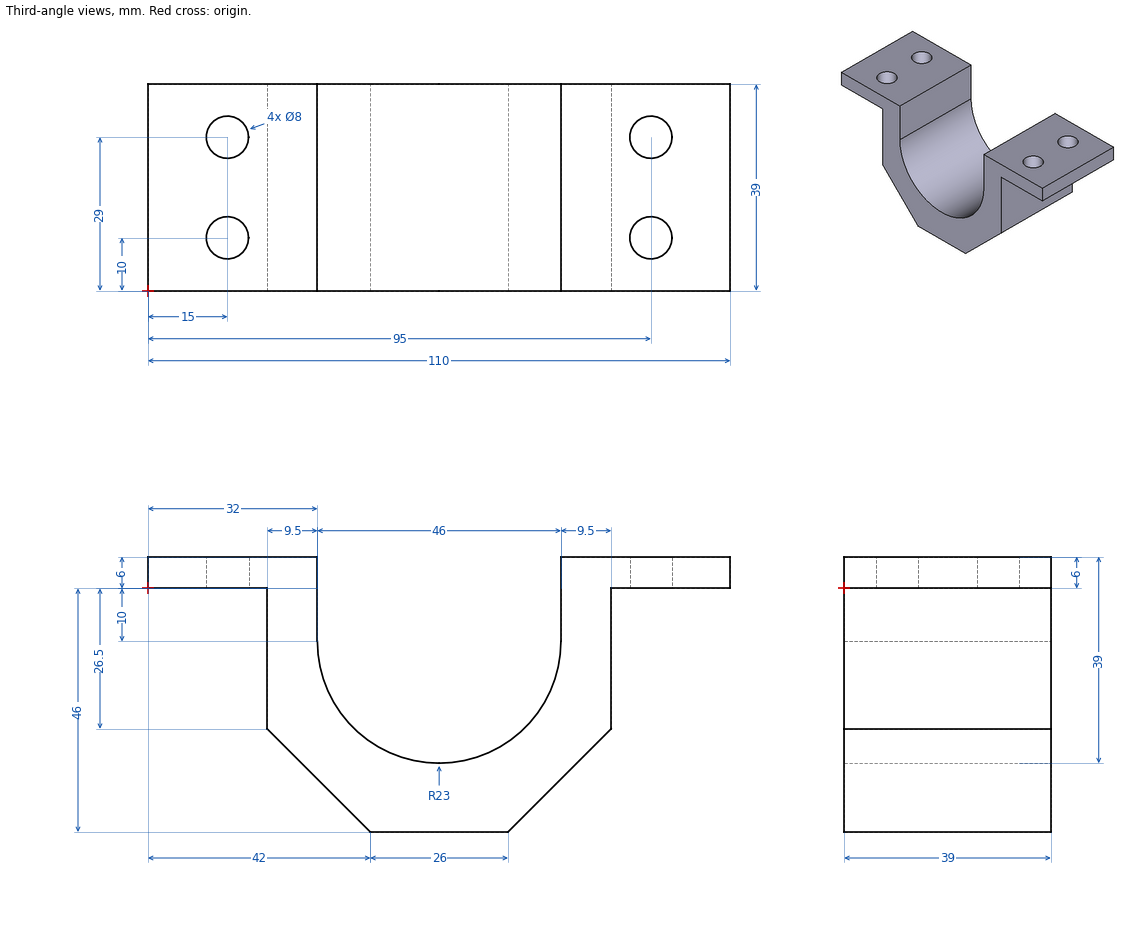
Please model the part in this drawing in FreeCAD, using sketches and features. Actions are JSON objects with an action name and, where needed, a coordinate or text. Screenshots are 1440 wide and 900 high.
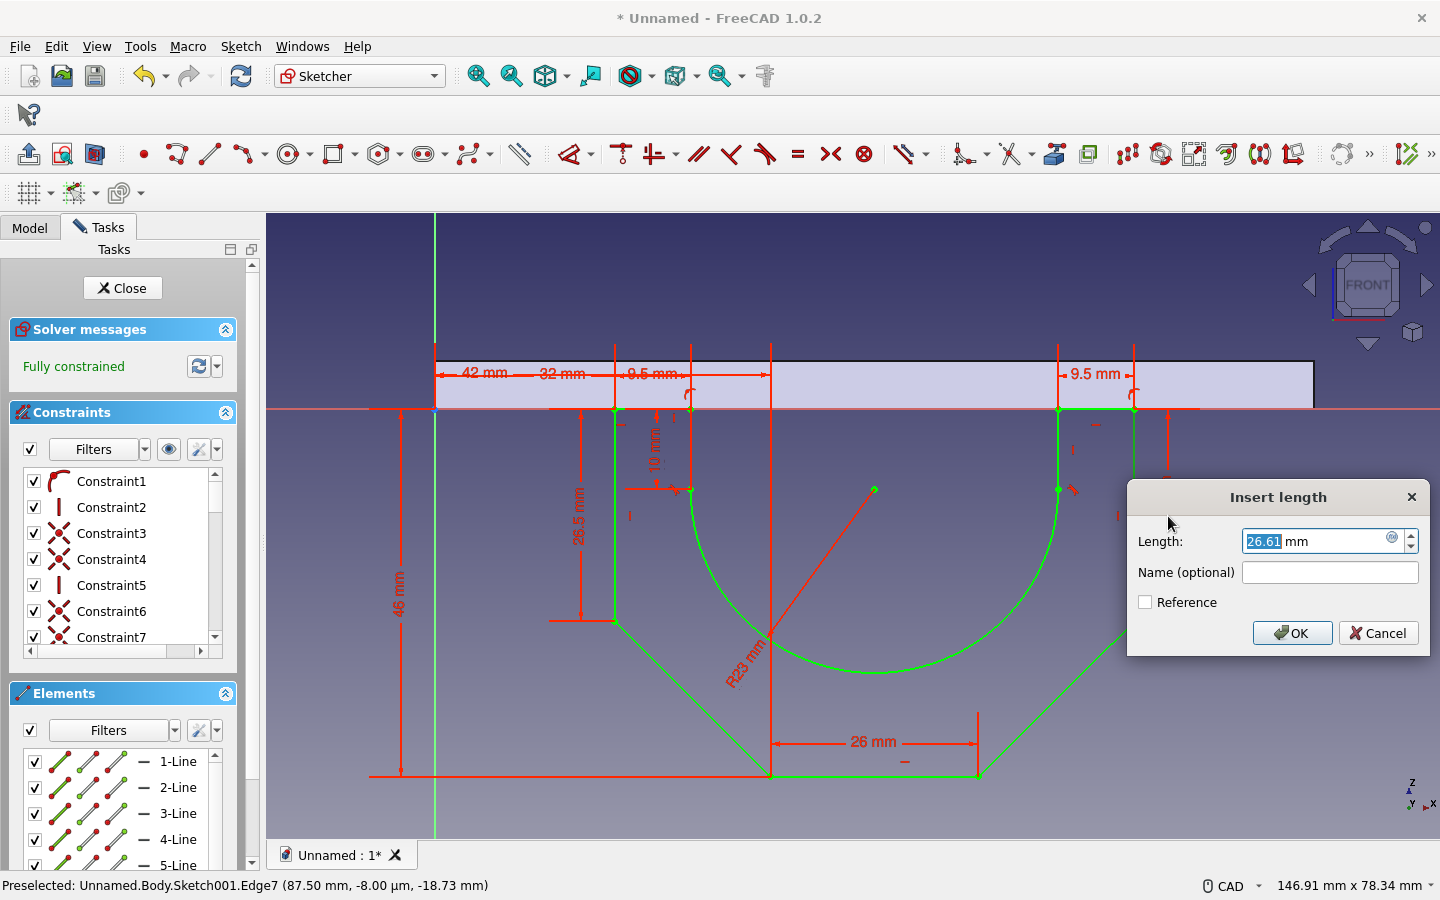
{"action": "type", "text": "26.5"}
{"action": "key", "text": "Return"}
{"action": "key", "text": "Escape"}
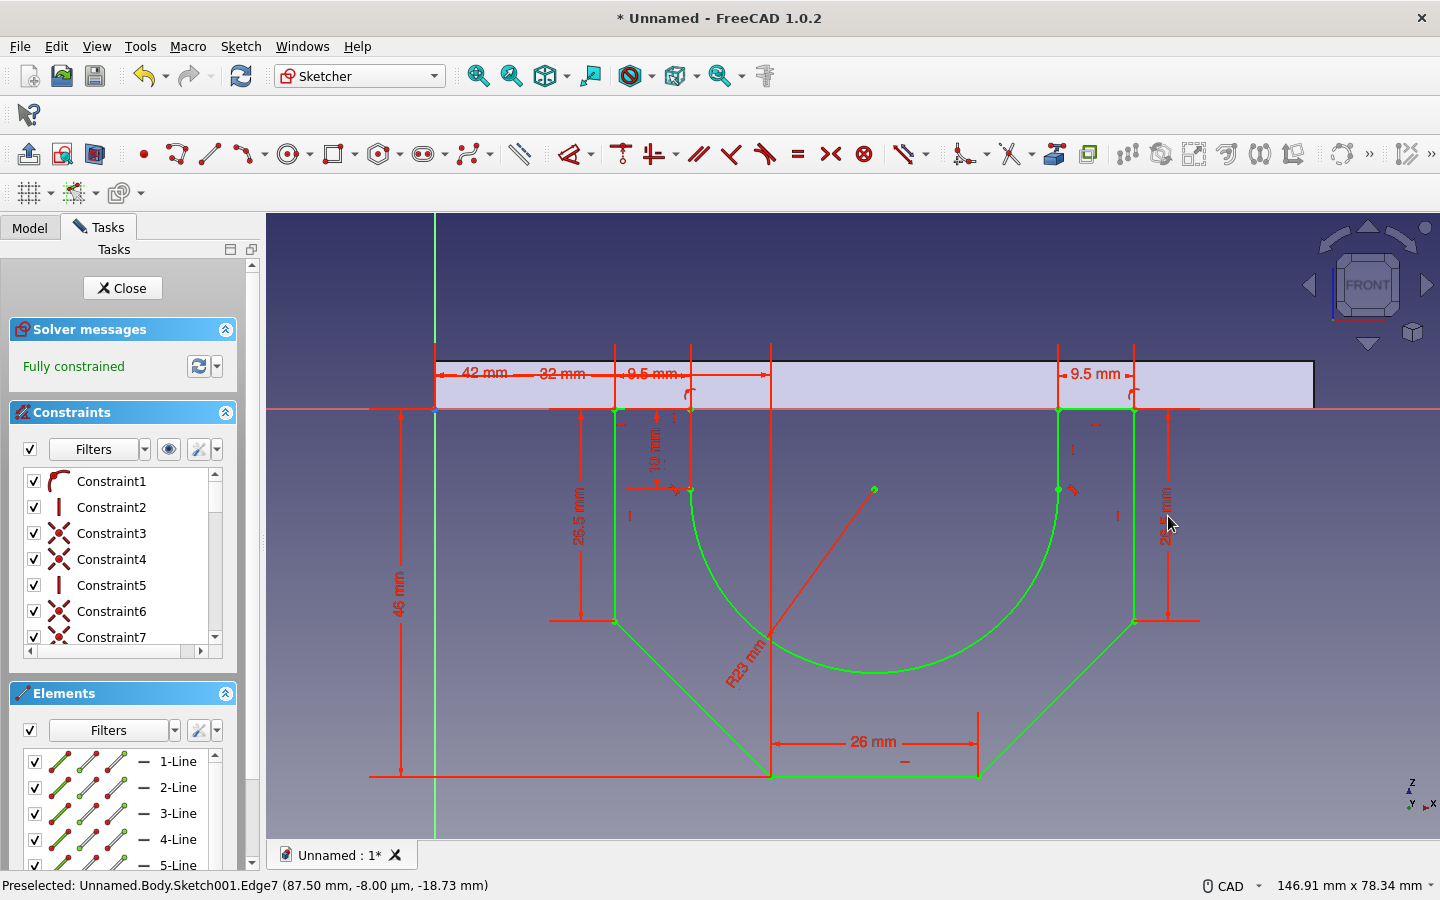
{"action": "left_click", "coordinate": [123, 288]}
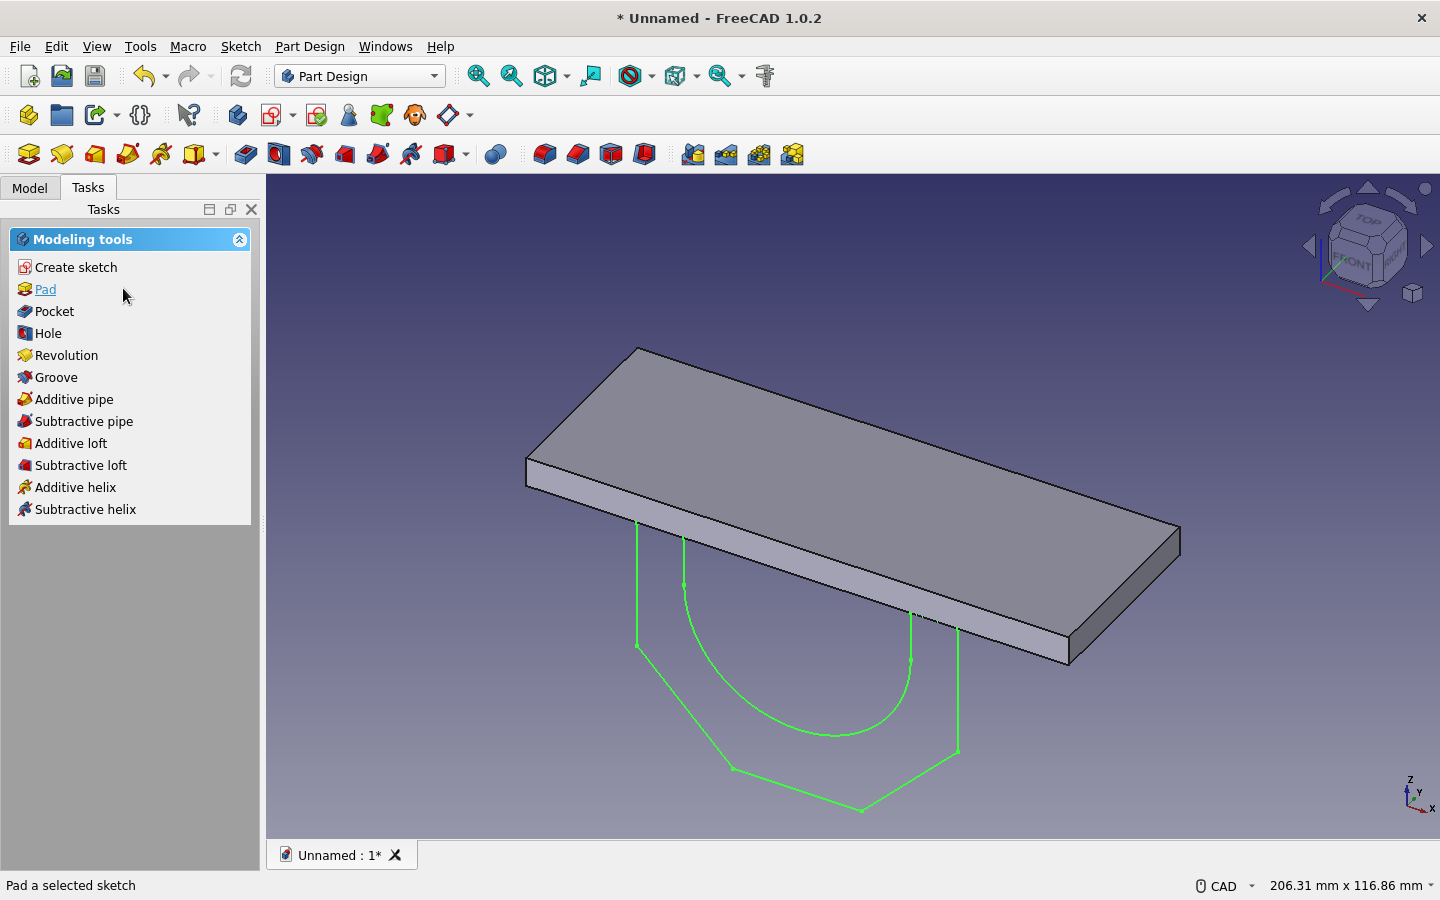
{"action": "left_click", "coordinate": [29, 154]}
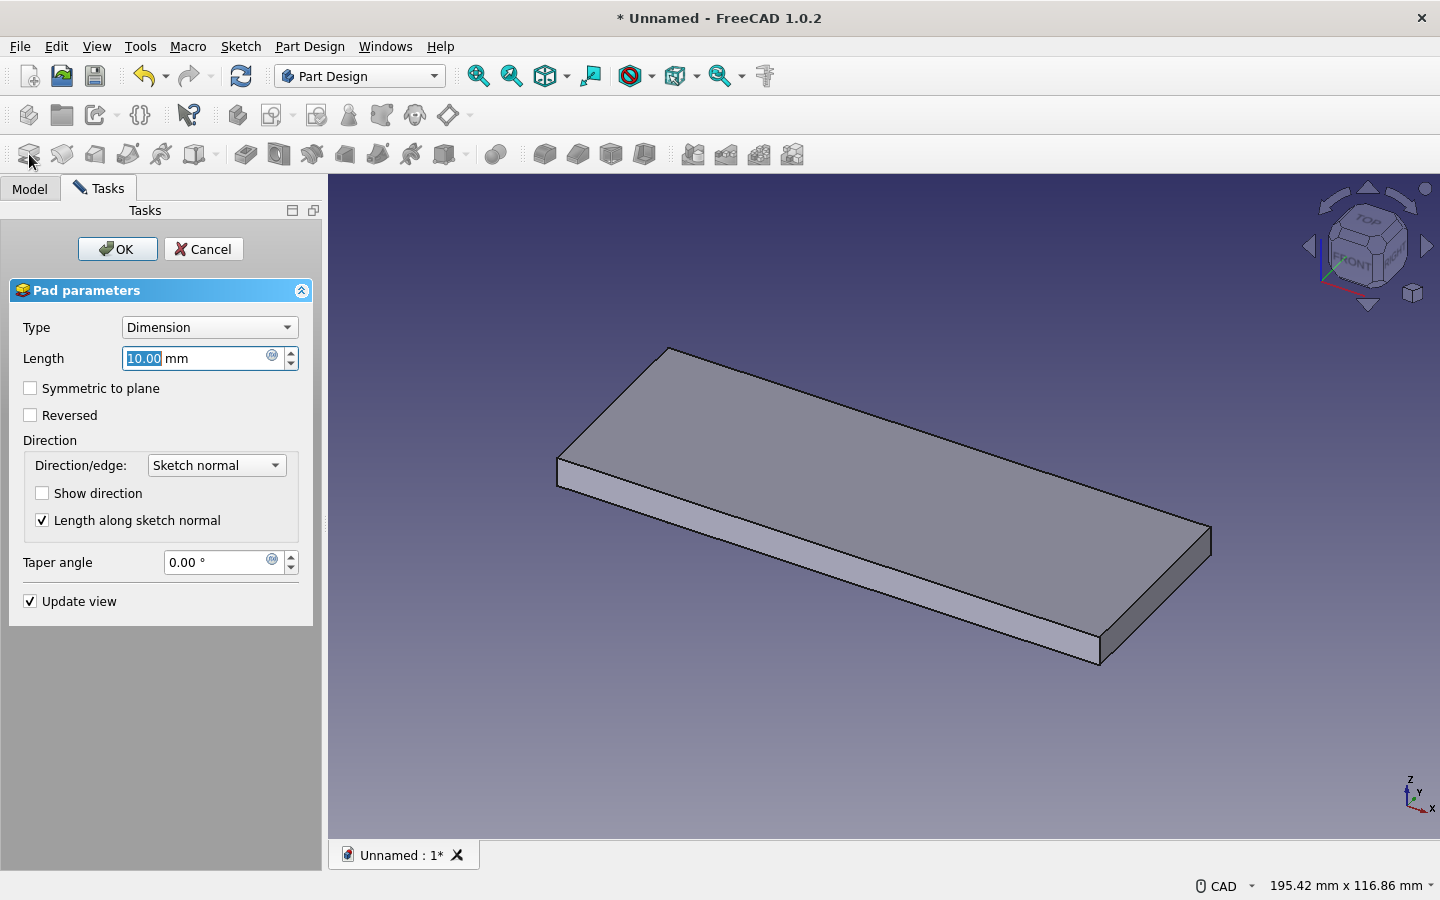
{"action": "type", "text": "39"}
{"action": "key", "text": "Tab"}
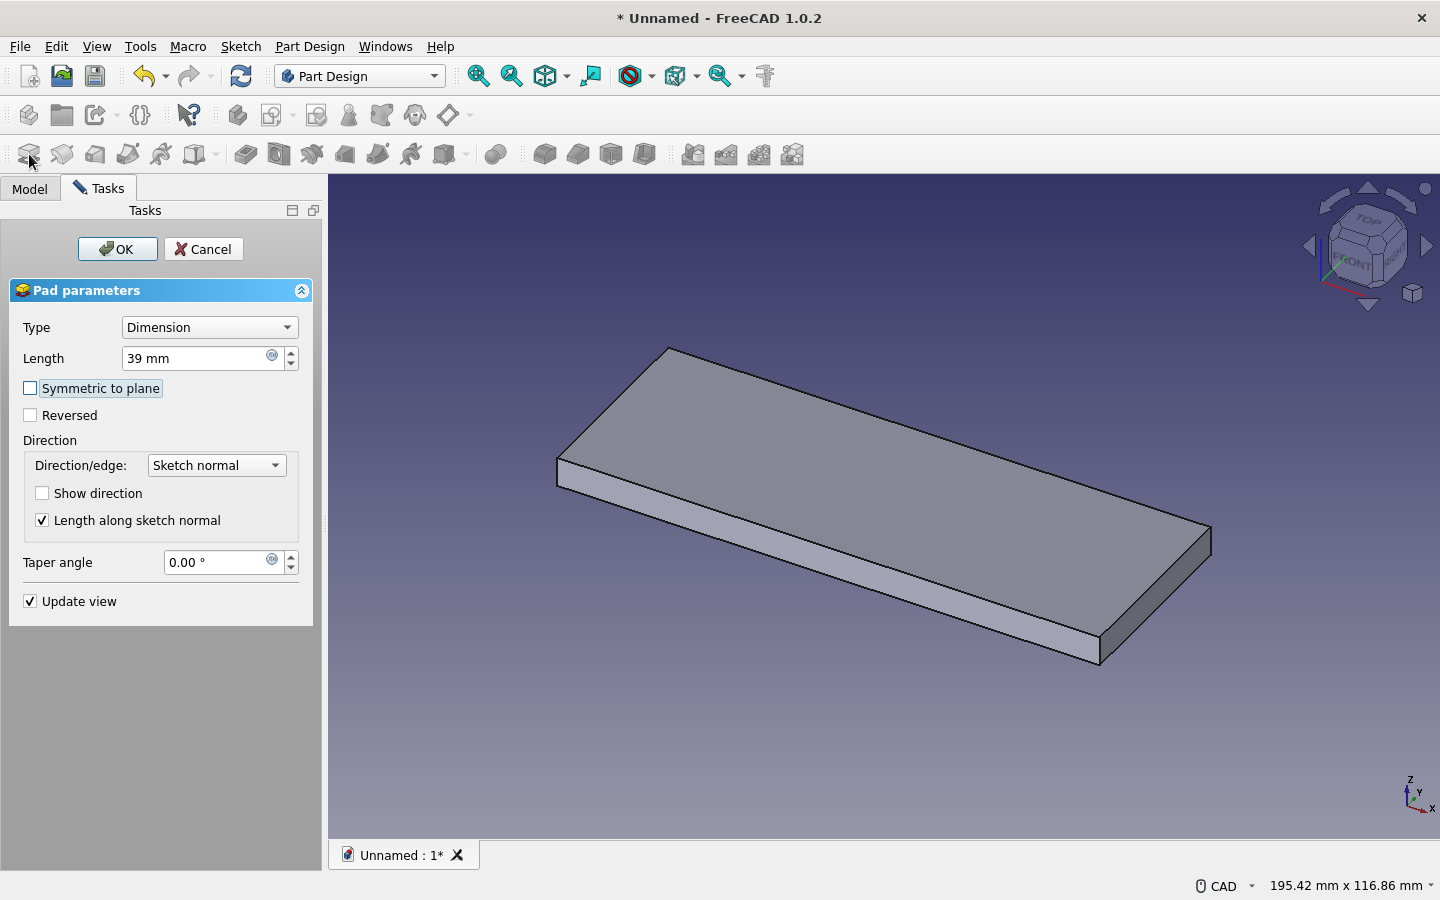
{"action": "left_click", "coordinate": [31, 415]}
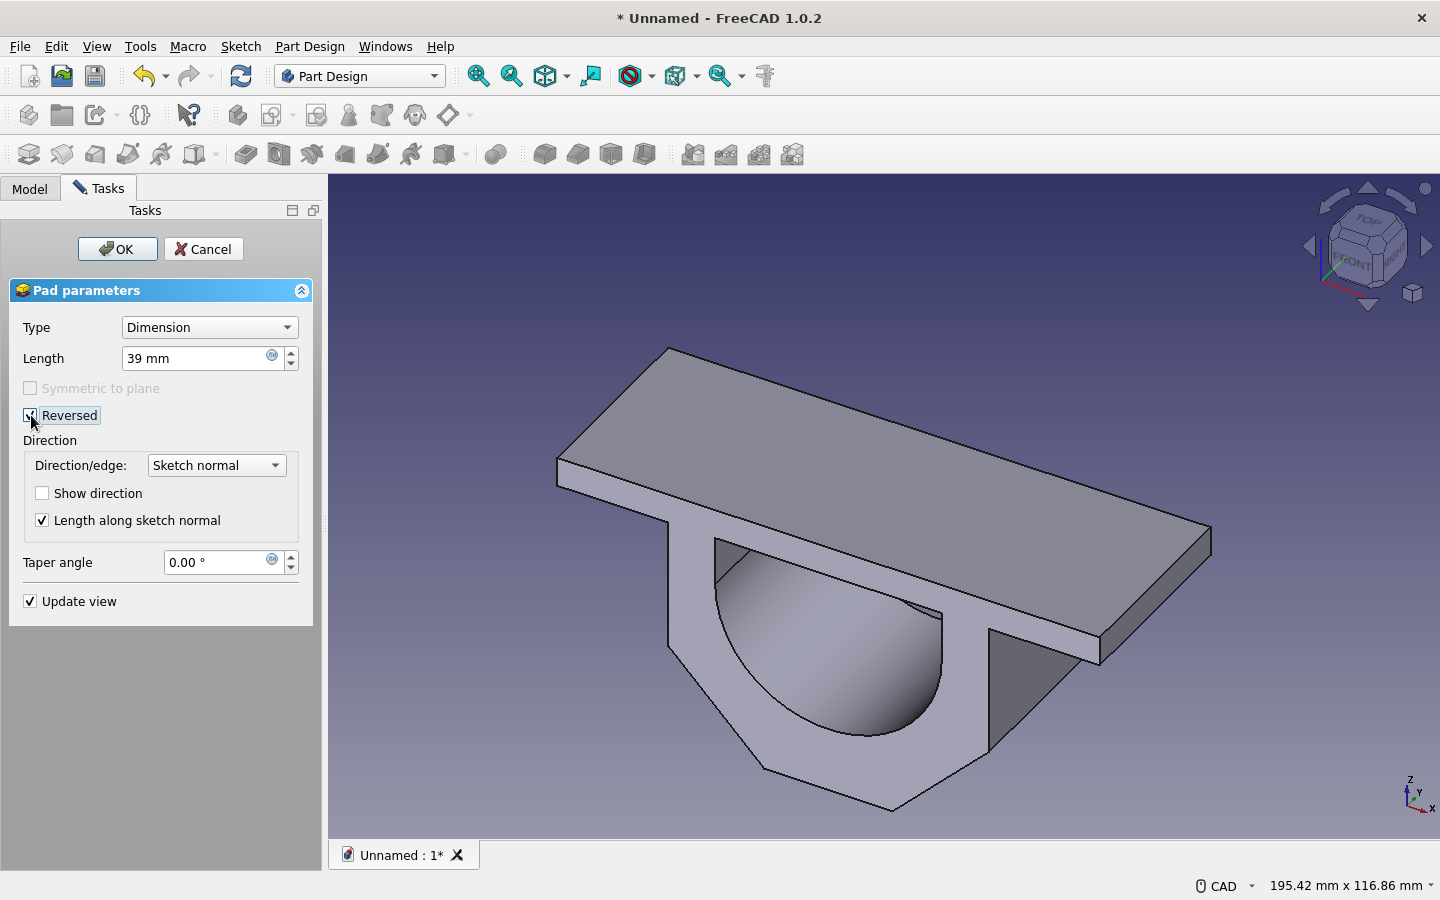
{"action": "left_click", "coordinate": [118, 249]}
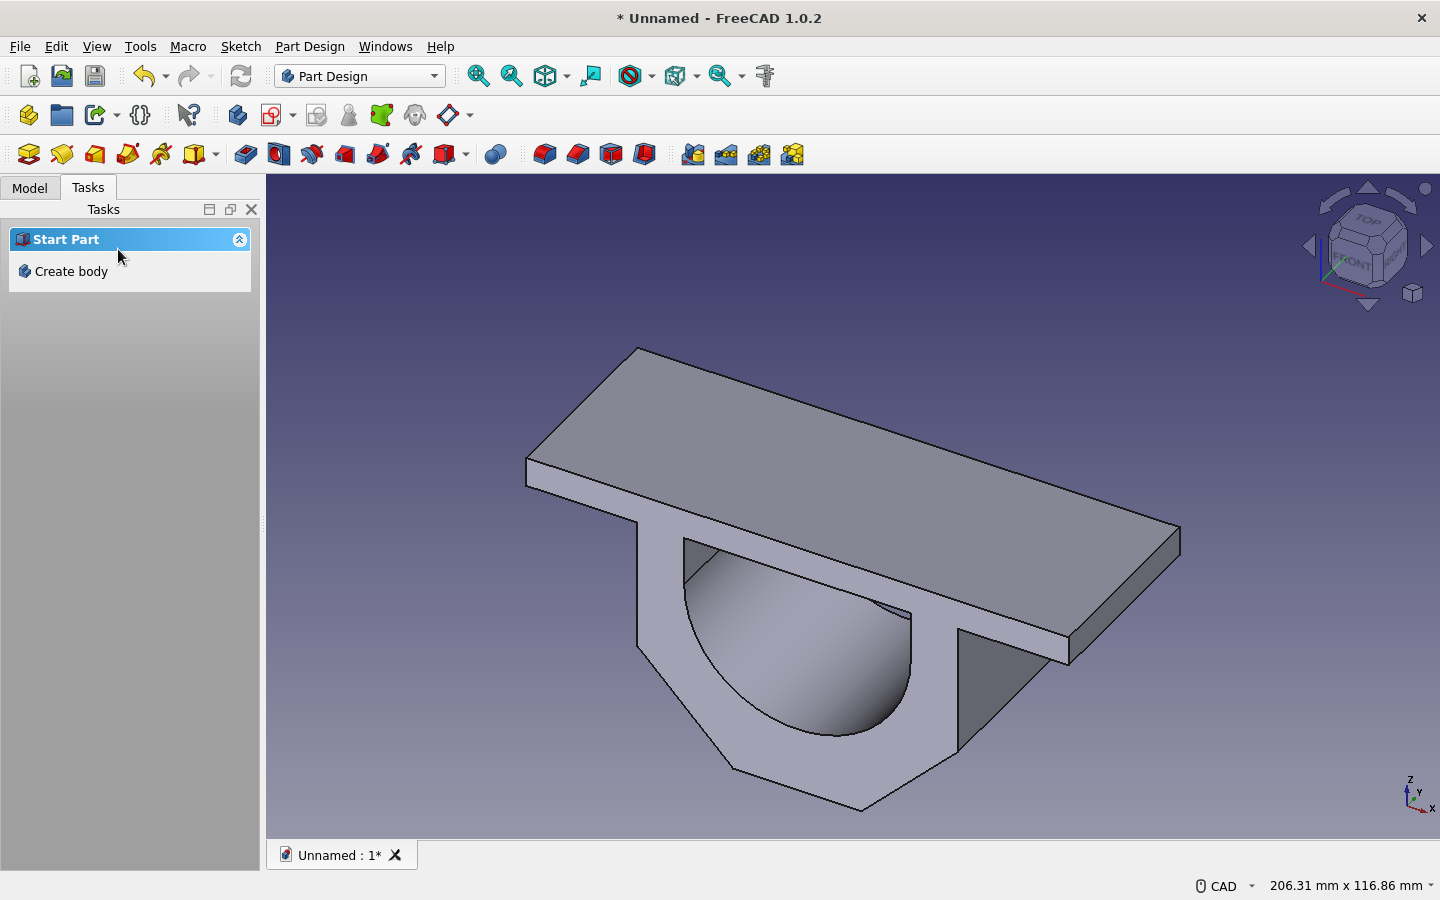
{"action": "left_click", "coordinate": [479, 76]}